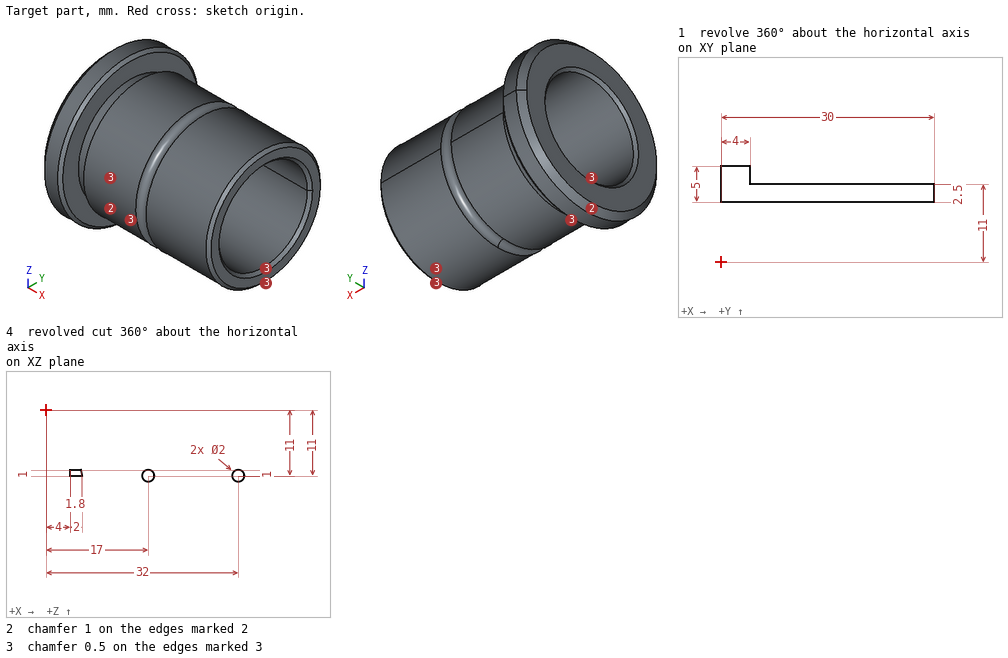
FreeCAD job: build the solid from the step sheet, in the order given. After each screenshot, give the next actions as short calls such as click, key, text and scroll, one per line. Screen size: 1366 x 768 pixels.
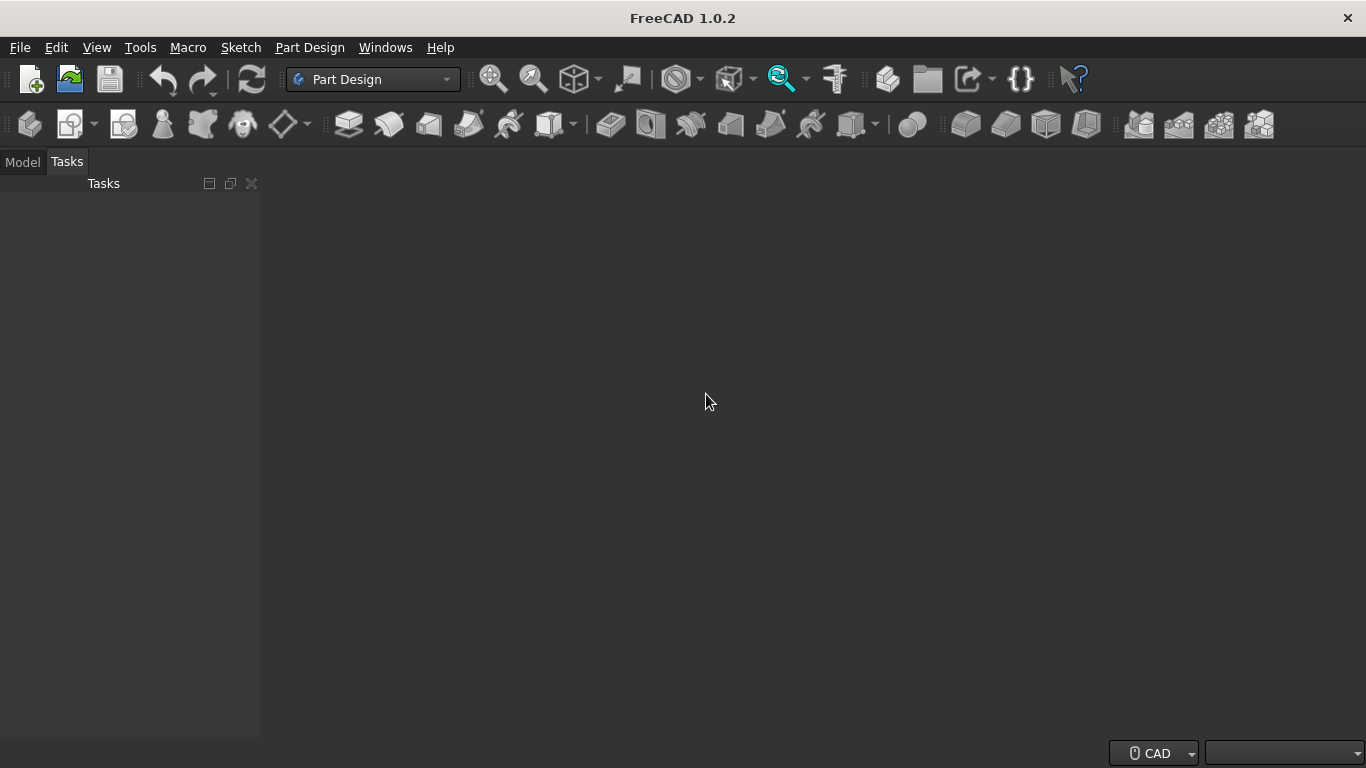
click(30, 80)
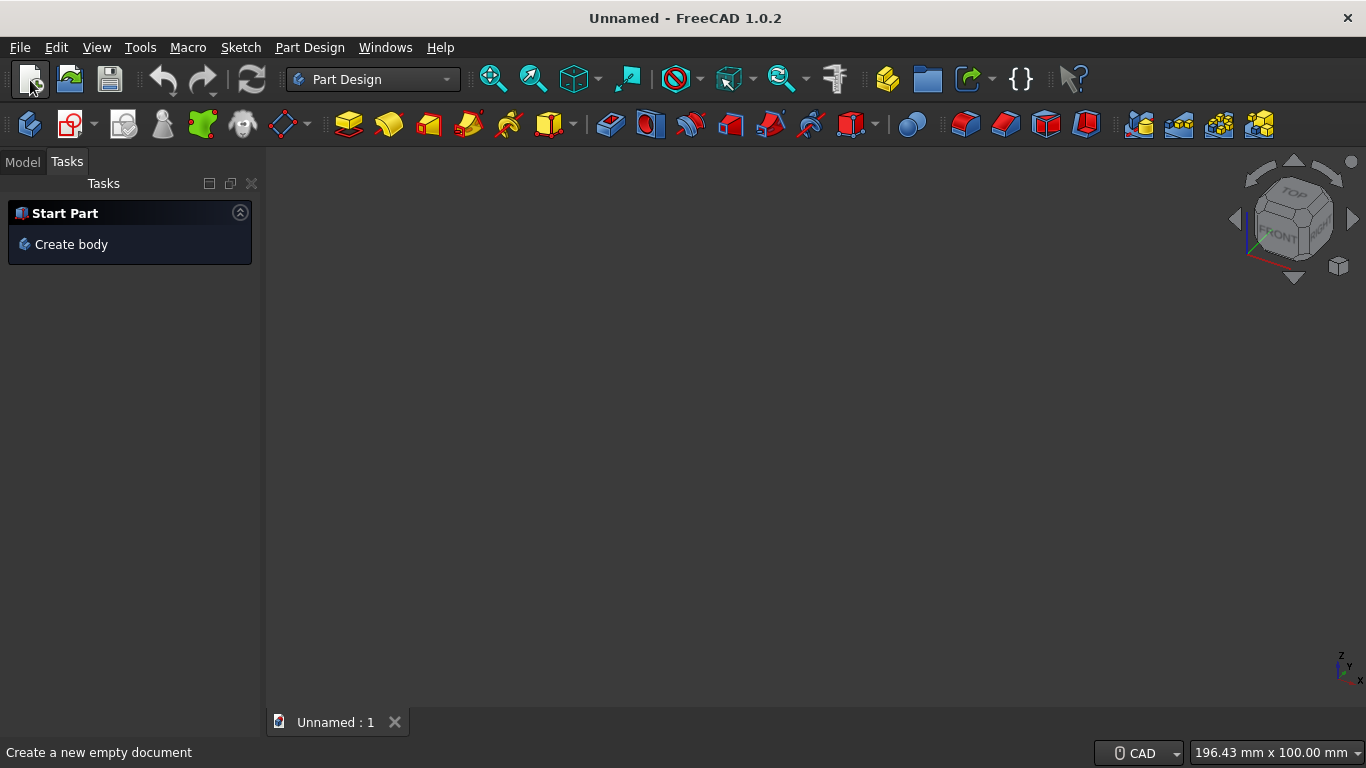
click(70, 124)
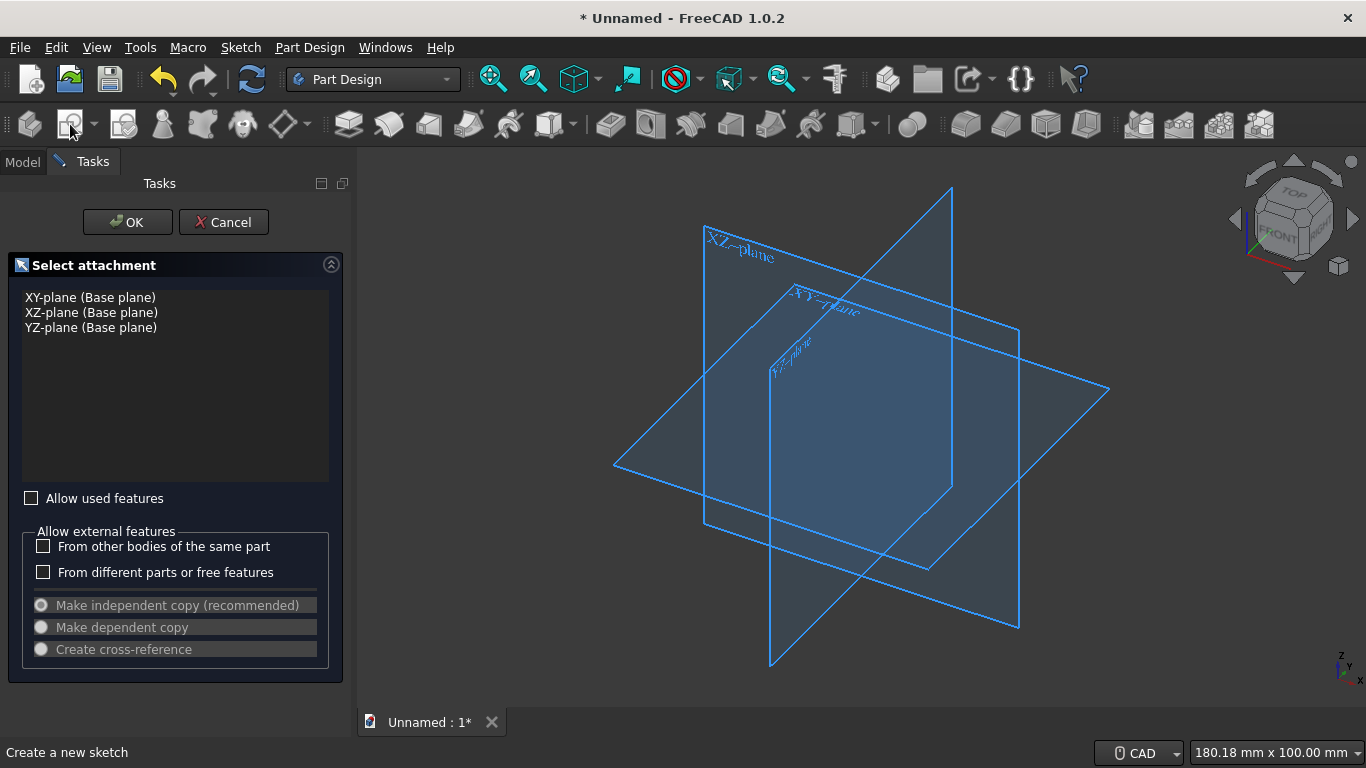
click(82, 298)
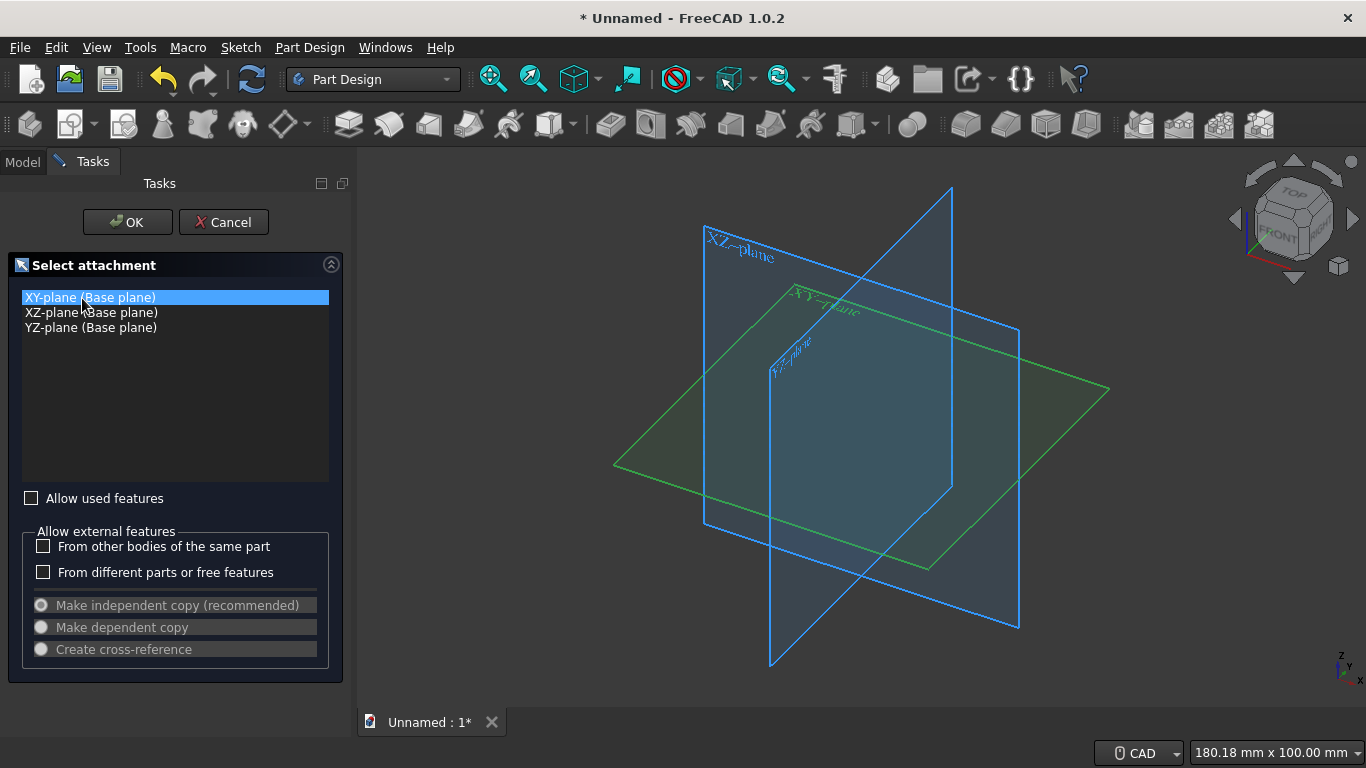
click(128, 222)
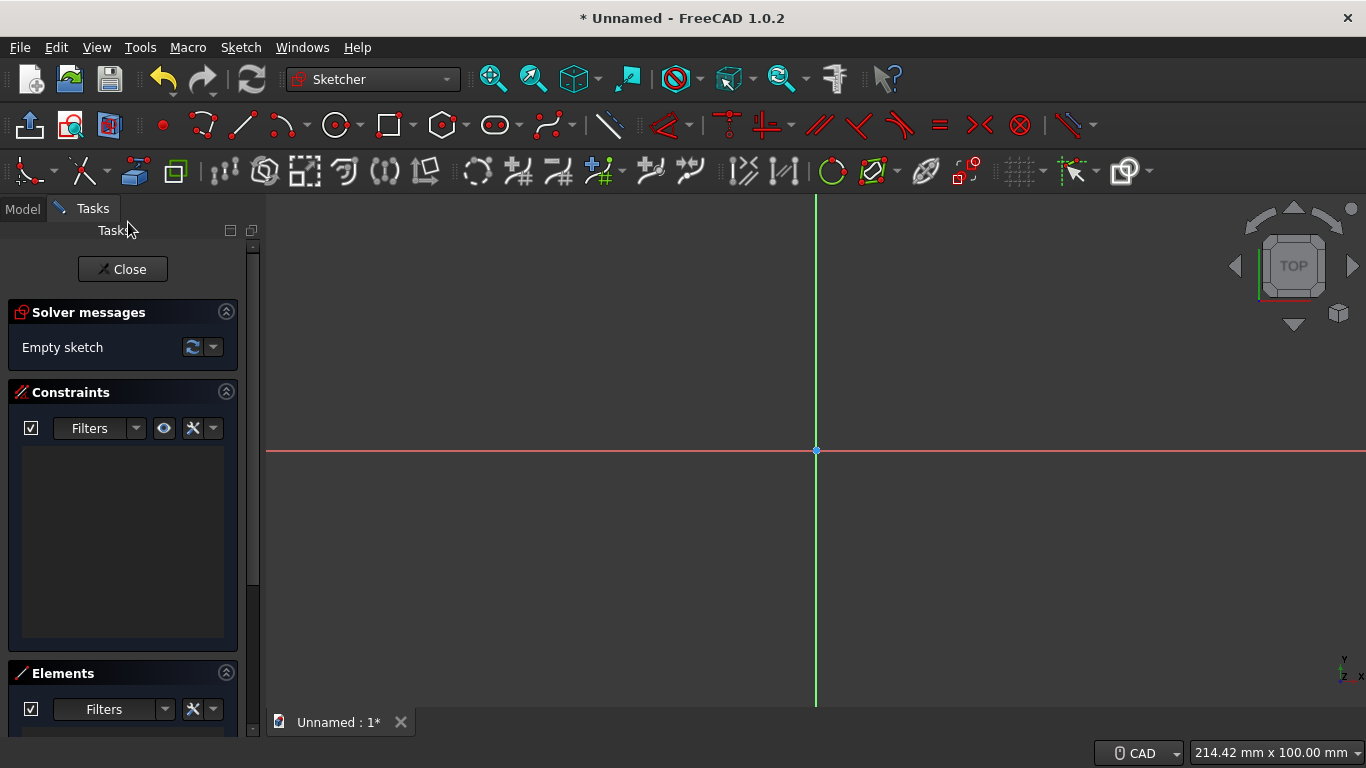
scroll(941, 405, up, 7)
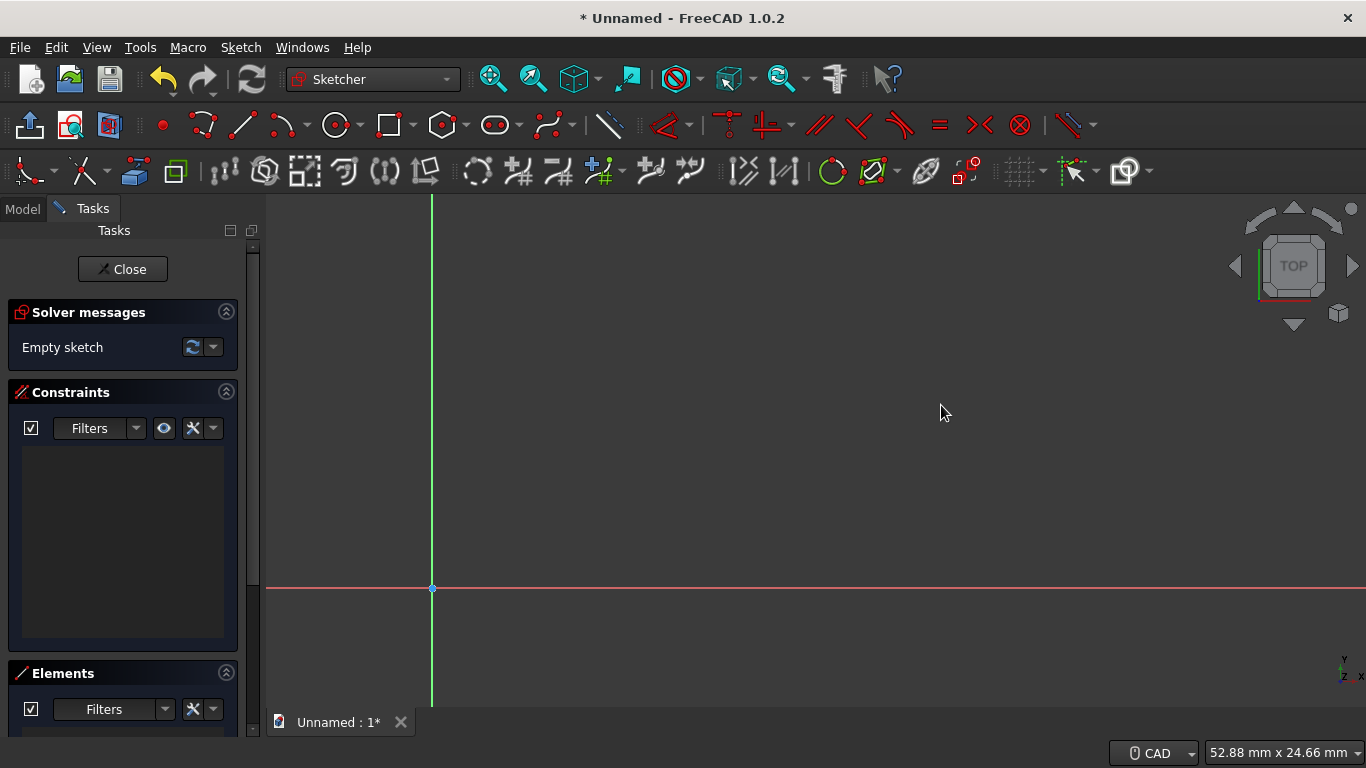
click(204, 126)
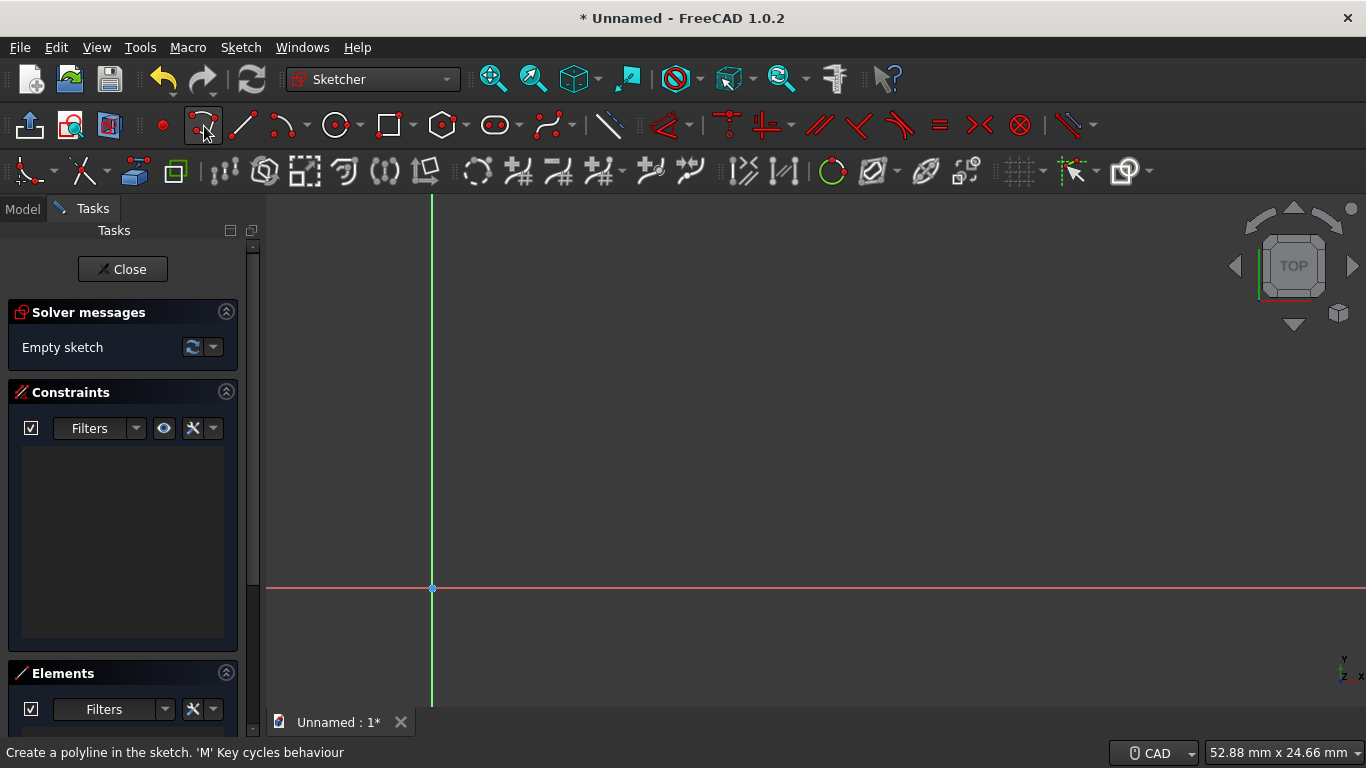
click(432, 411)
click(1056, 411)
click(1056, 359)
click(515, 359)
click(515, 307)
click(441, 307)
click(432, 412)
key(Escape)
key(Escape)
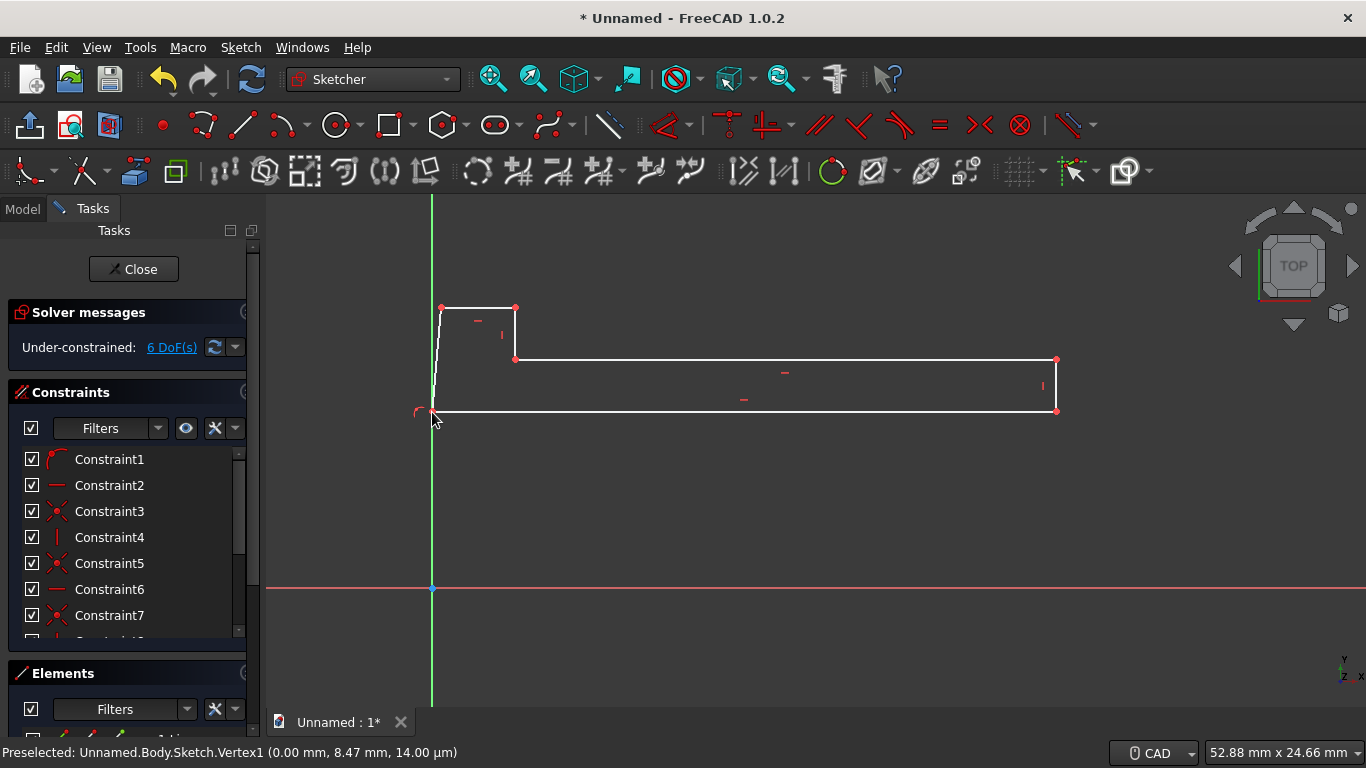
click(435, 381)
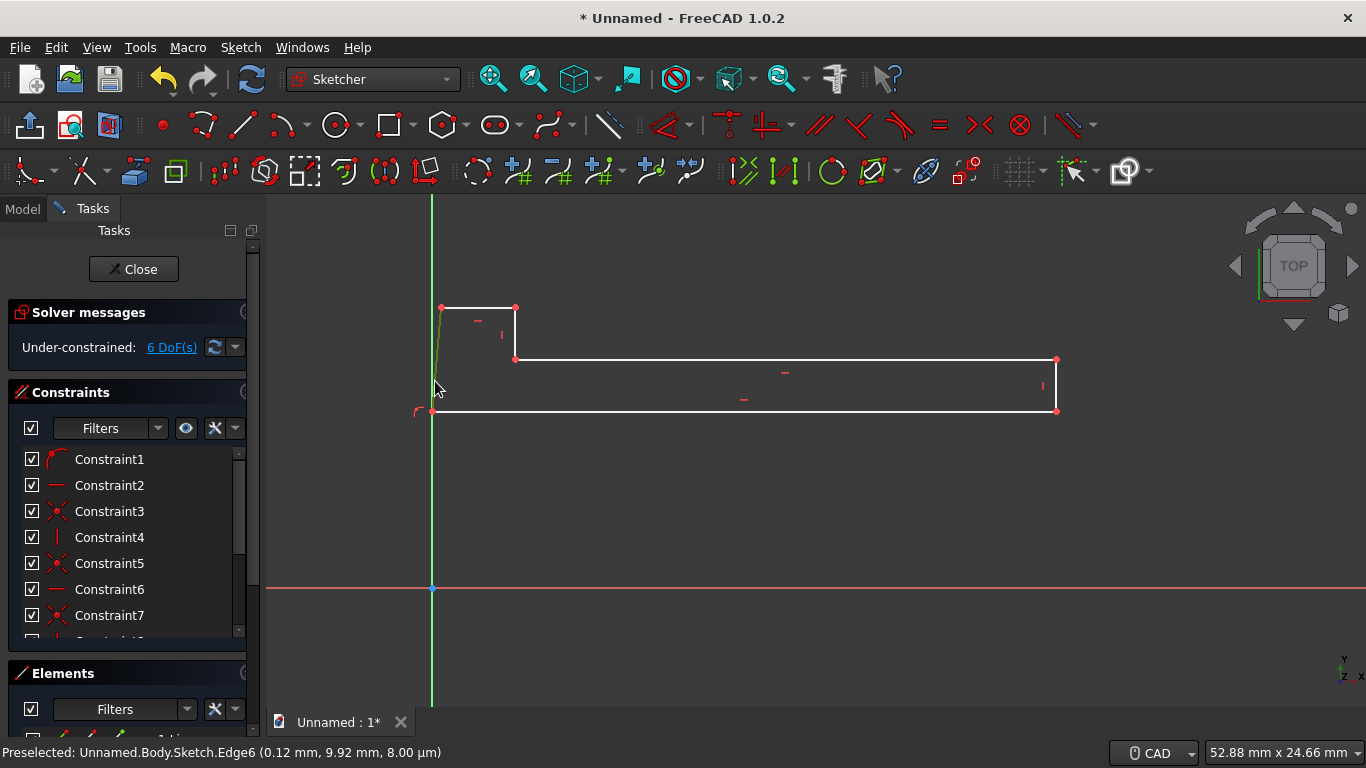
key(v)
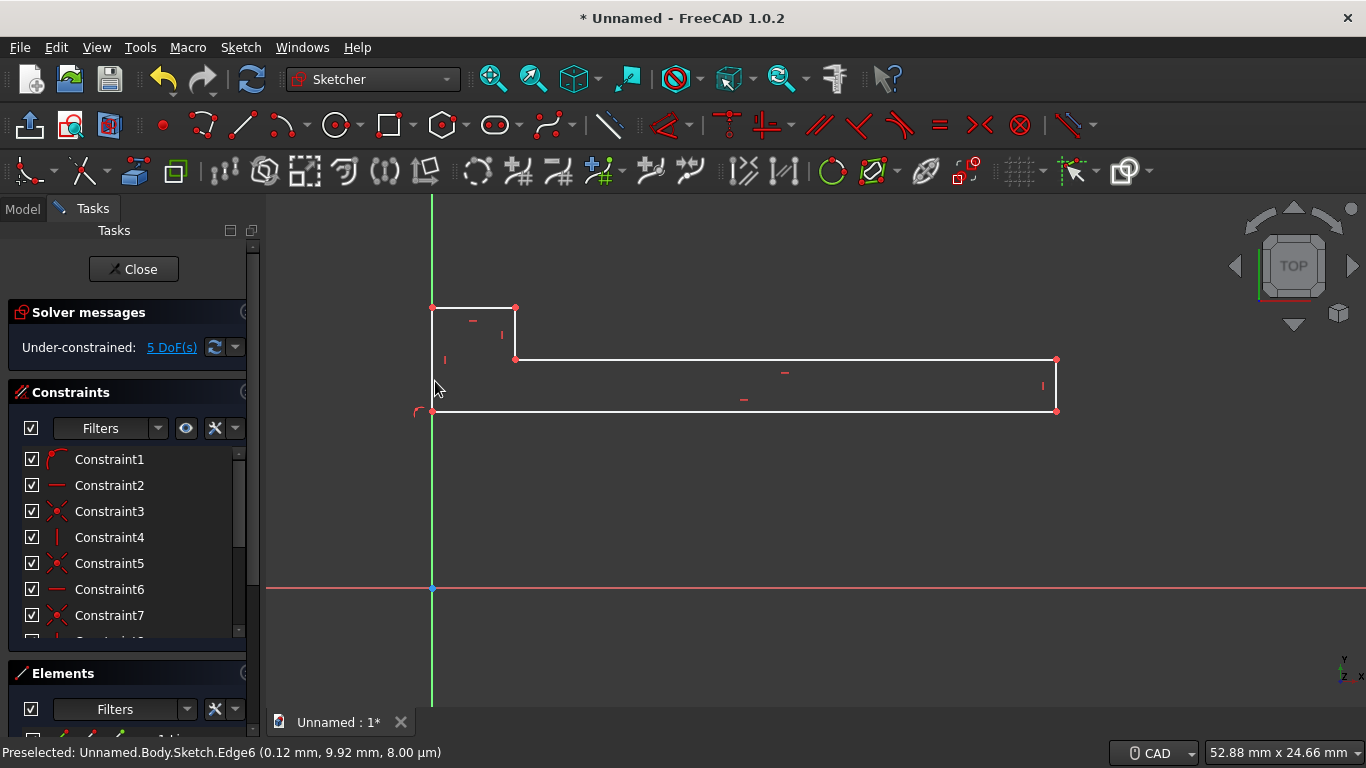
click(490, 308)